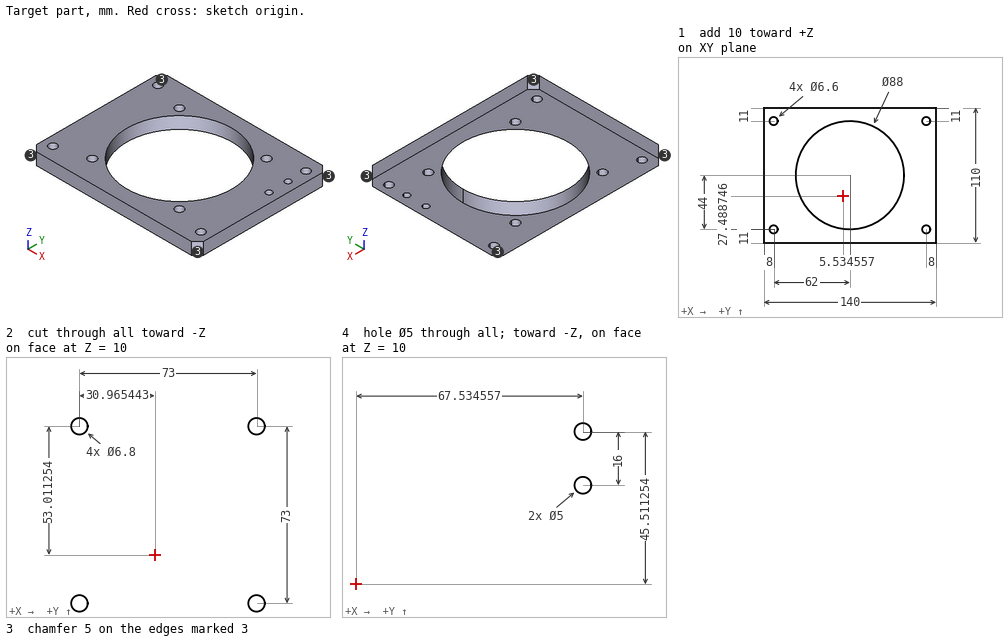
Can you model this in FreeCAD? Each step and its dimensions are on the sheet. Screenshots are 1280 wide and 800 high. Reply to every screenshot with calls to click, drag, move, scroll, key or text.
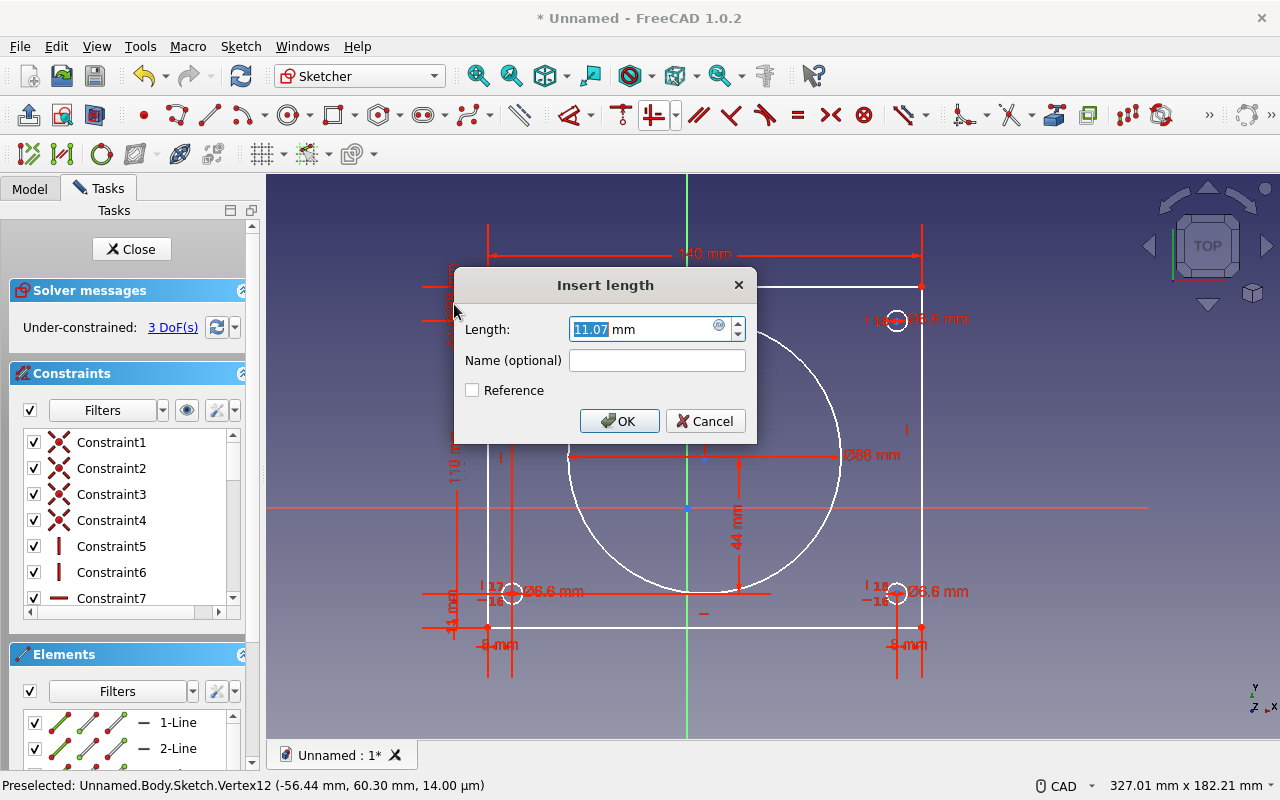
text(11)
key(Return)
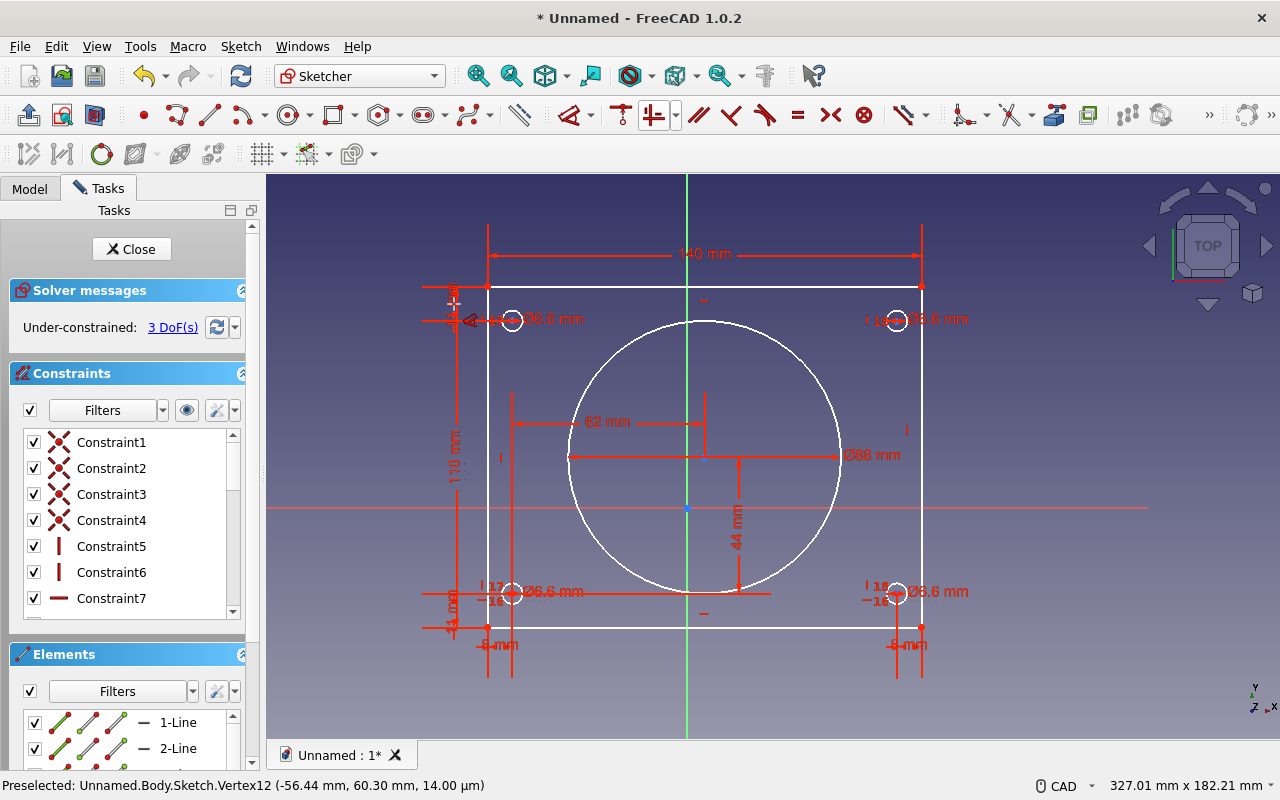
click(922, 287)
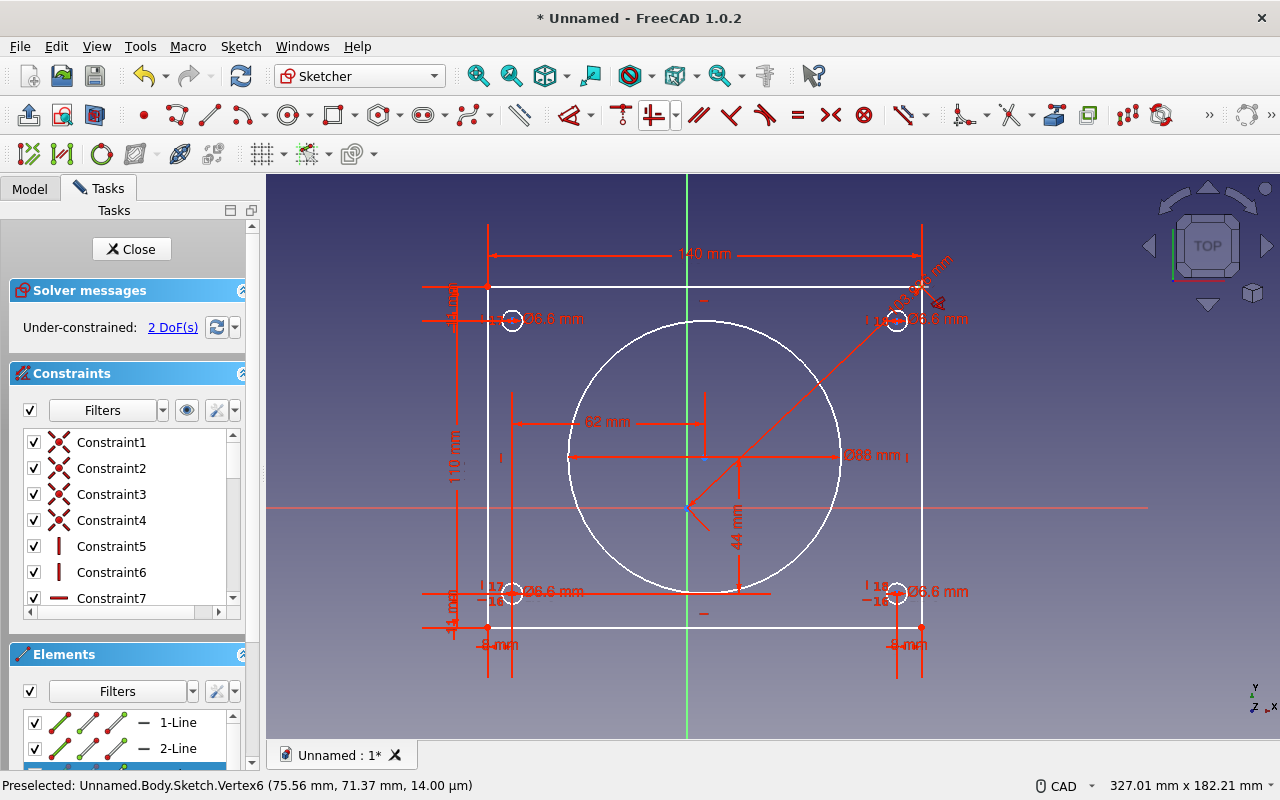
click(897, 321)
click(956, 304)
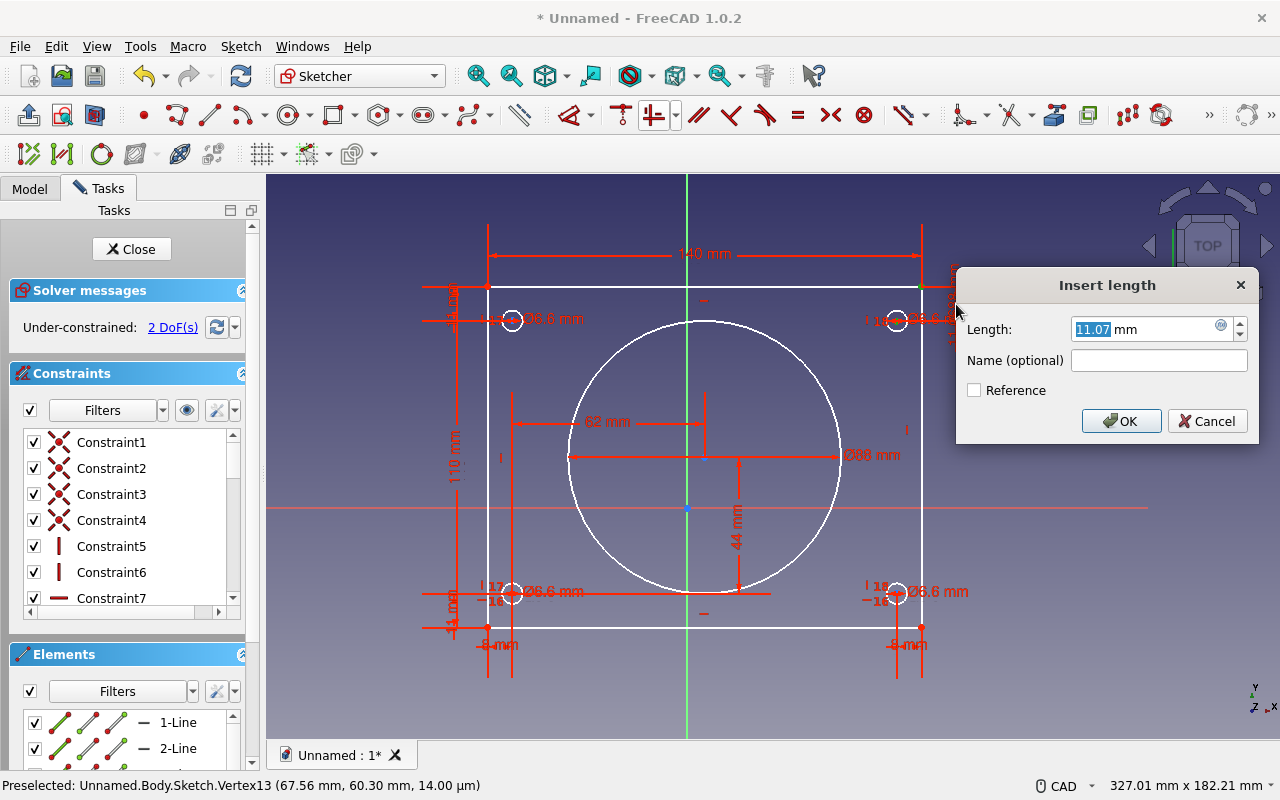
text(11)
key(Return)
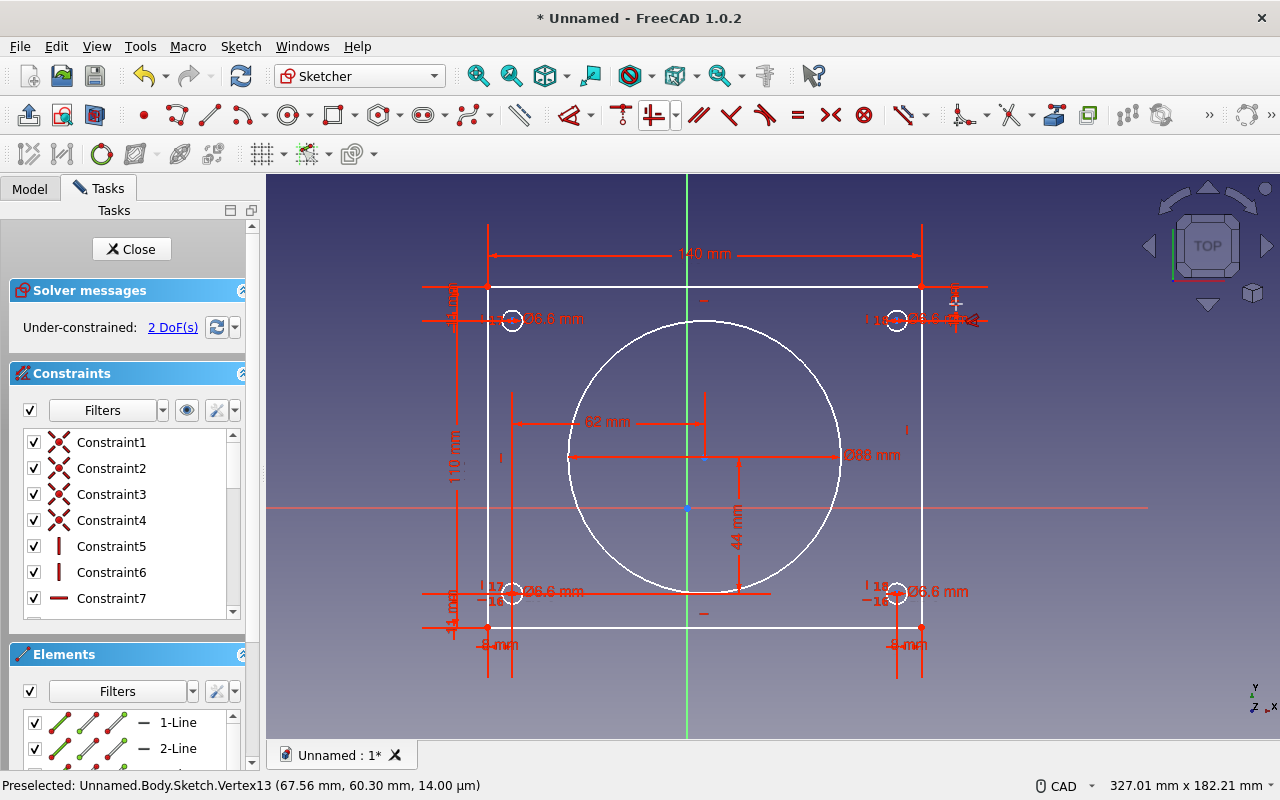
scroll(705, 457, up, 5)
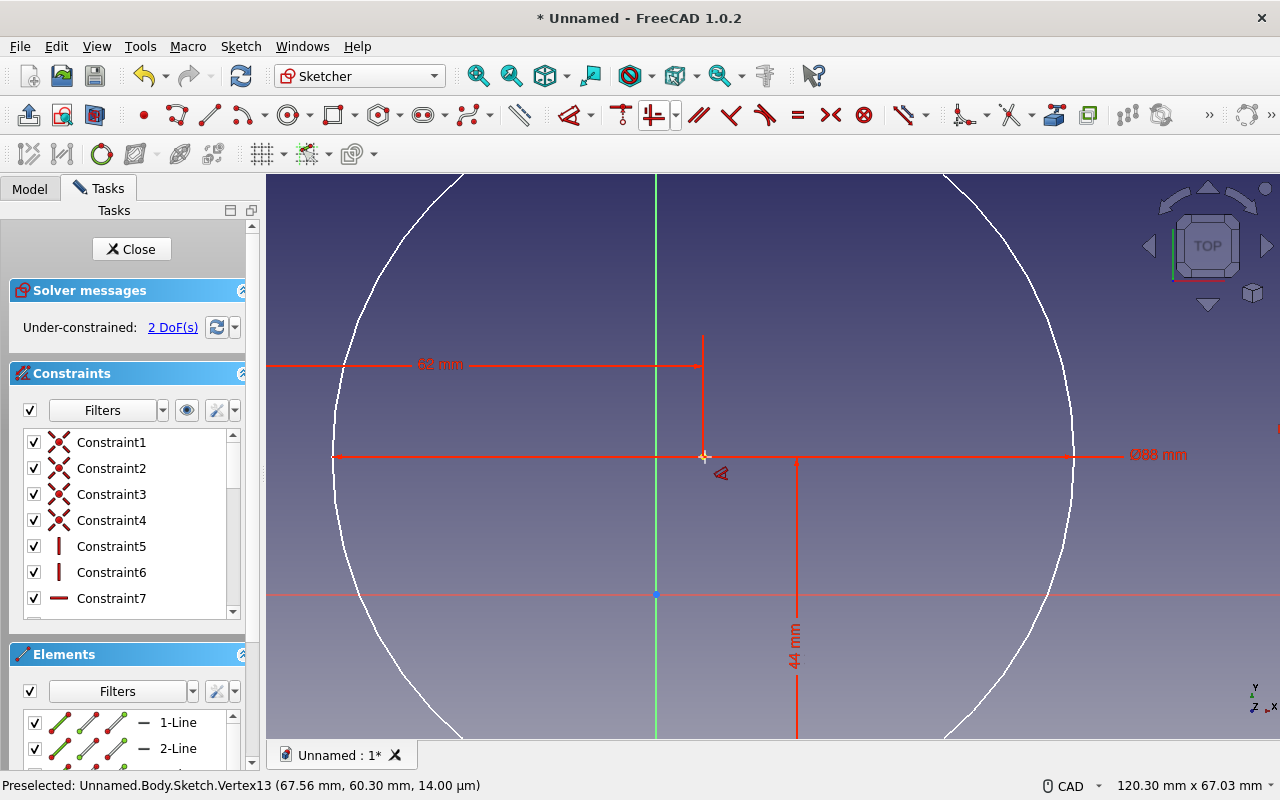
click(703, 457)
click(680, 629)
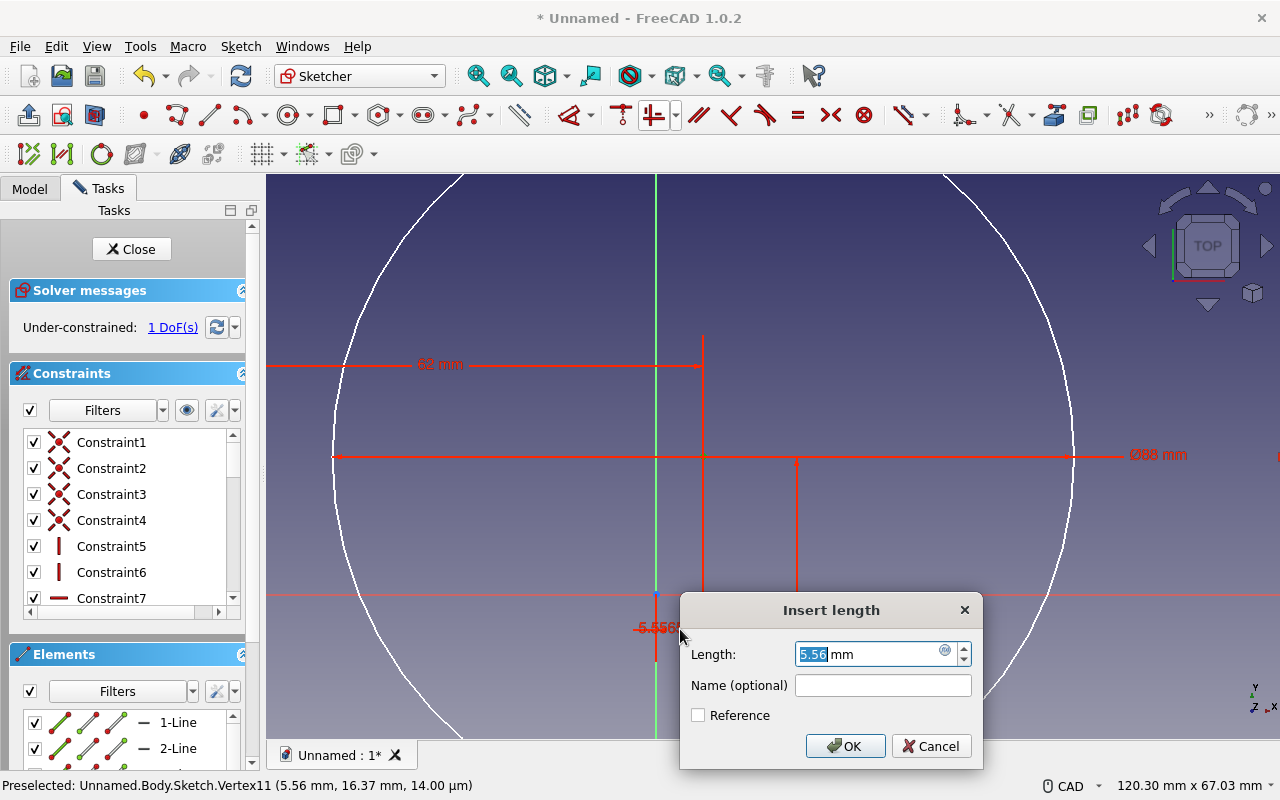
text(5.534557)
key(Return)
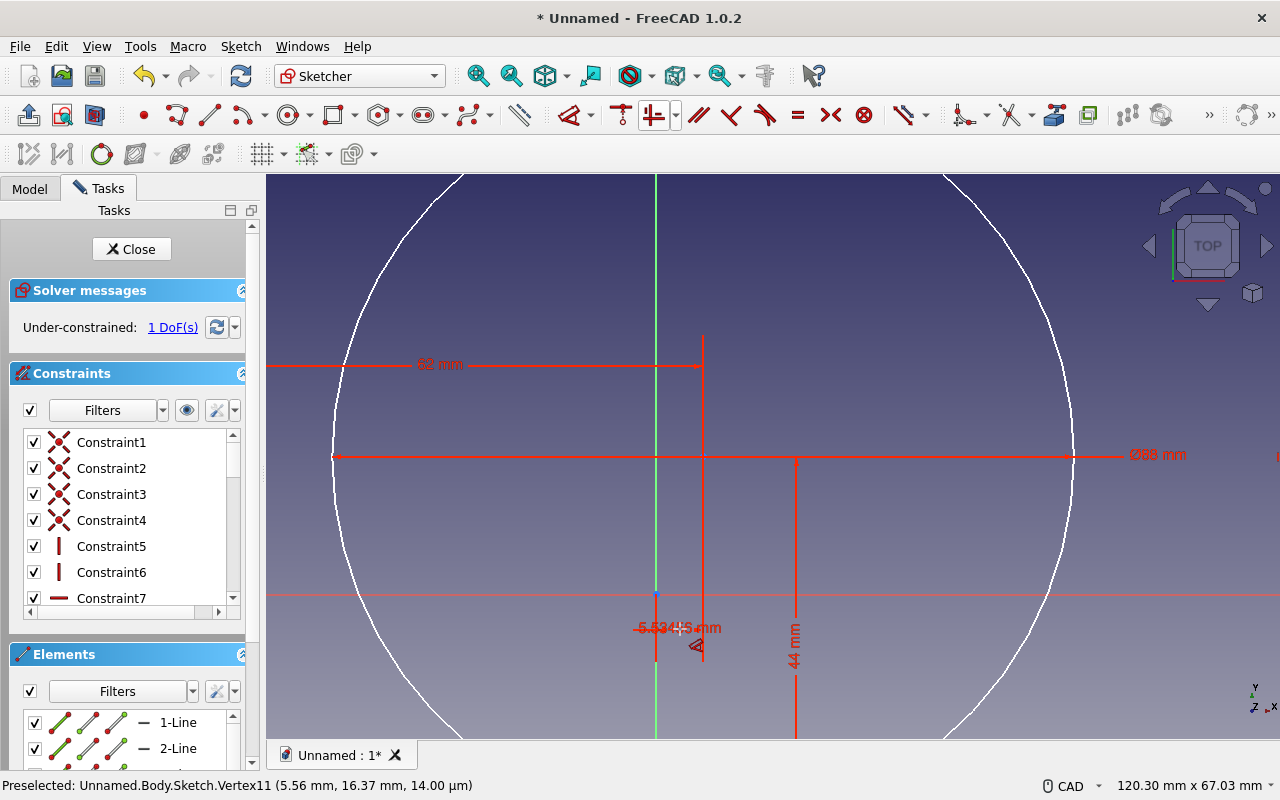
scroll(705, 457, down, 5)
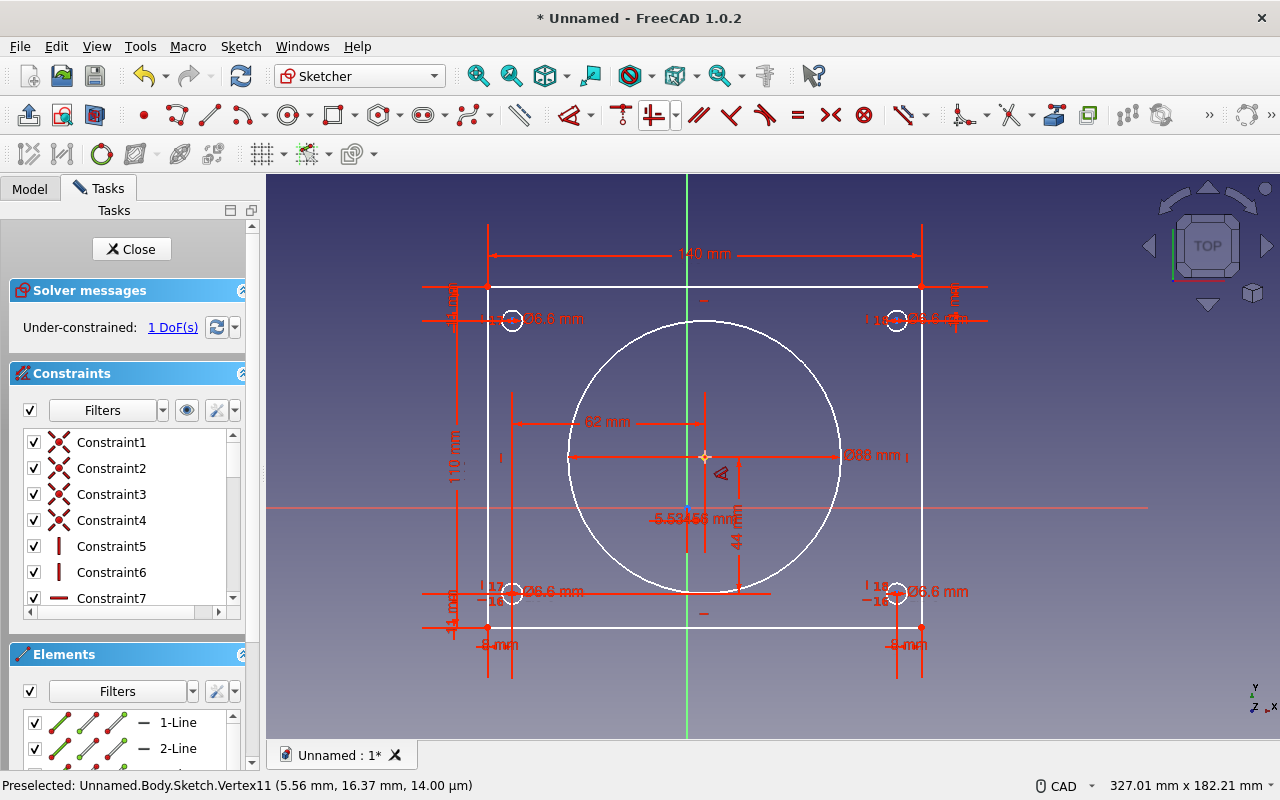
click(512, 594)
click(721, 551)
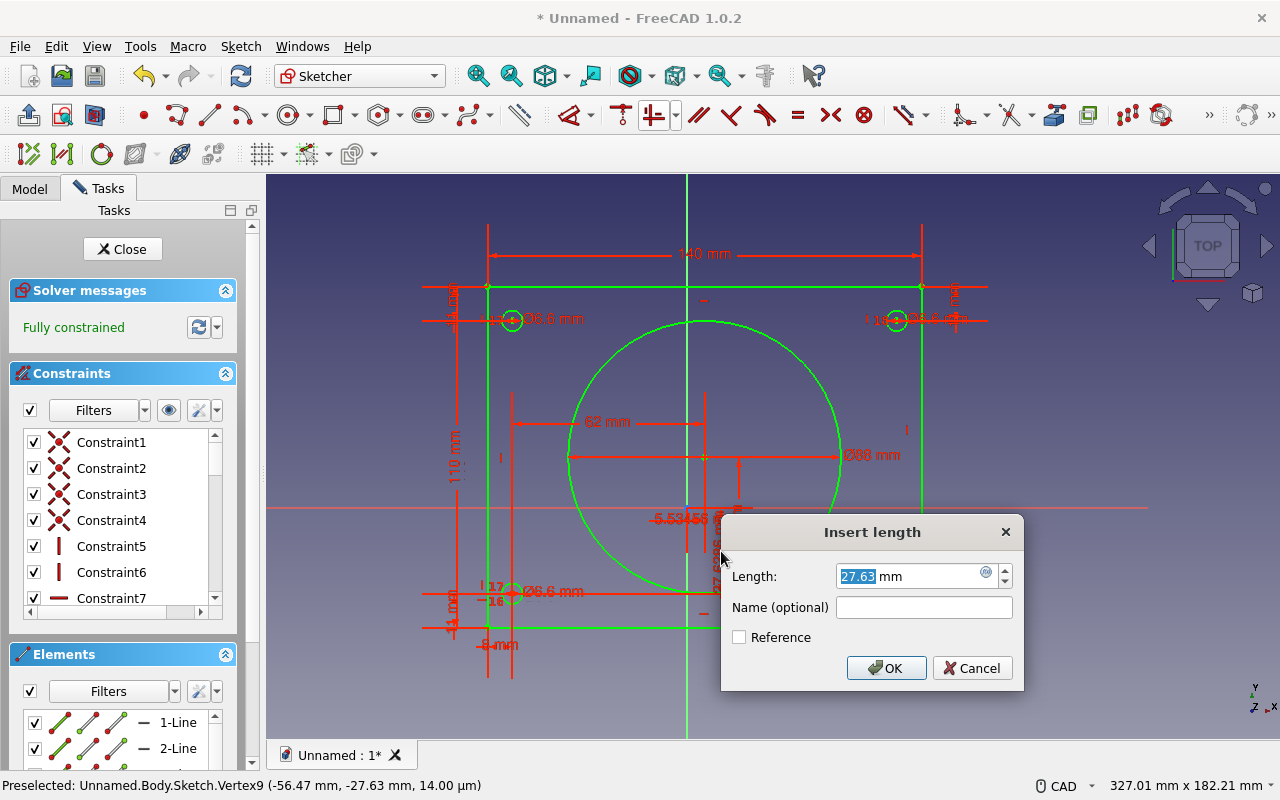
text(27.488746)
key(Return)
key(Escape)